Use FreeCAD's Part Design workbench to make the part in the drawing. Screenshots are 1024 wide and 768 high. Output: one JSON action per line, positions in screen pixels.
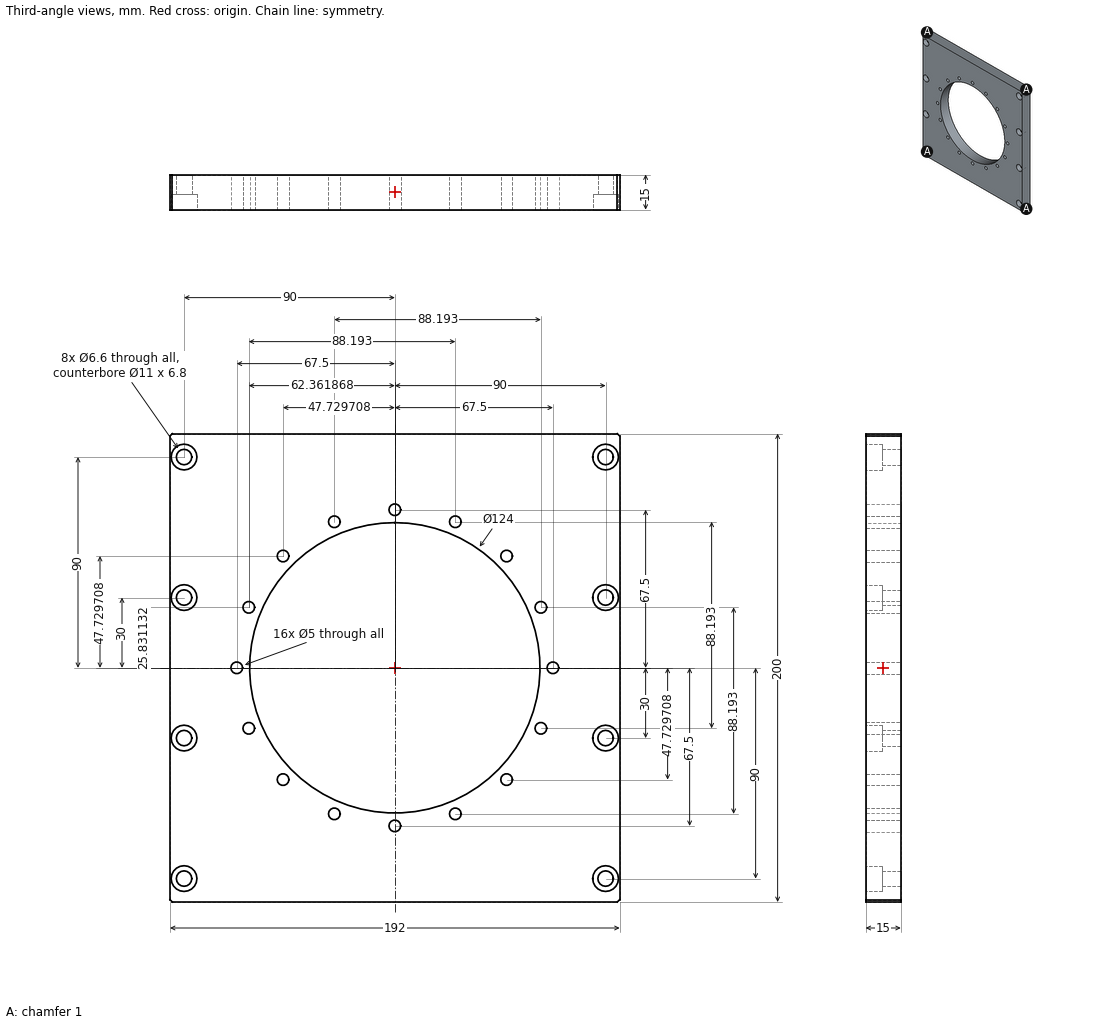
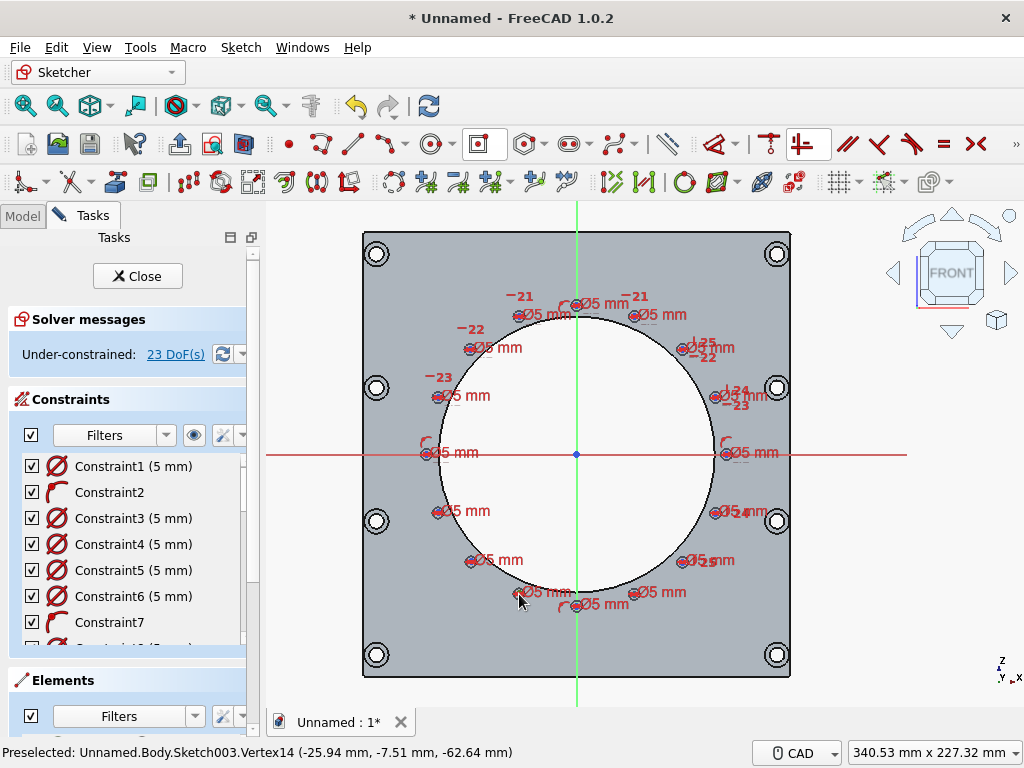
{"action": "key", "text": "h"}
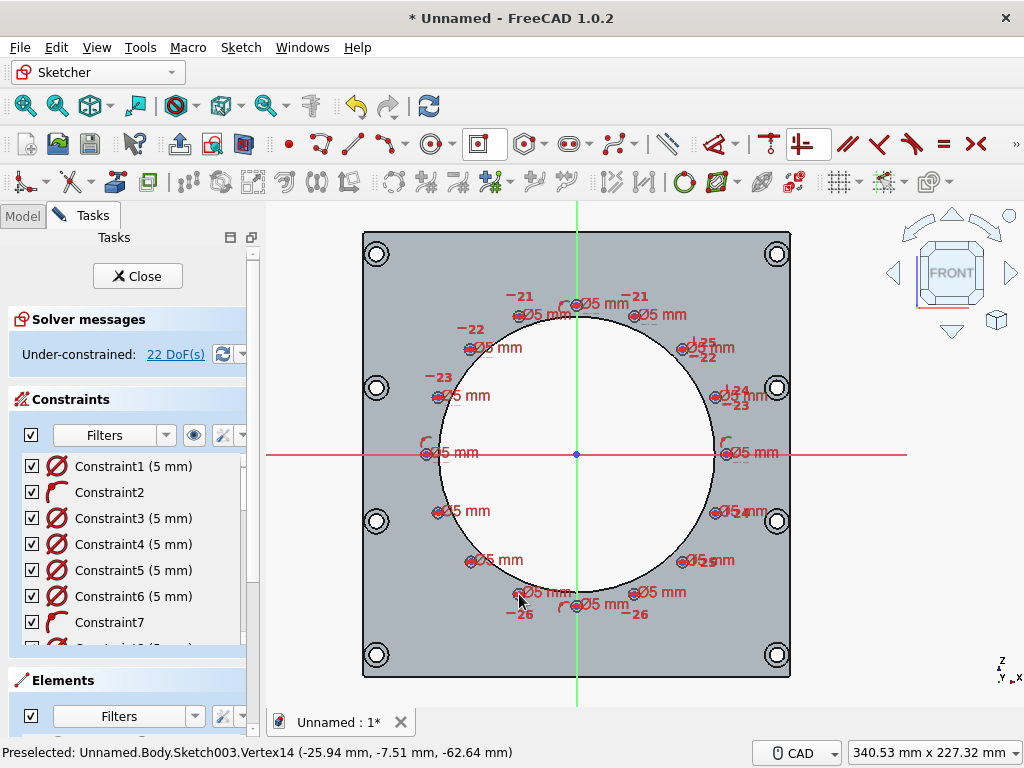
{"action": "left_click", "coordinate": [470, 350]}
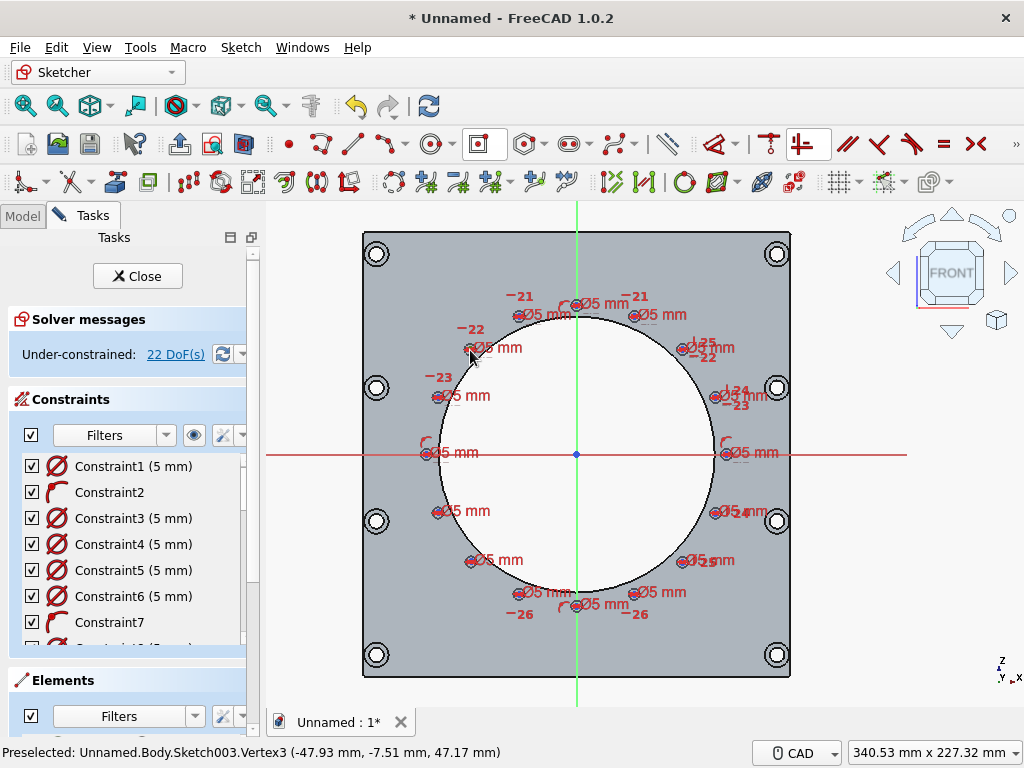
{"action": "left_click", "coordinate": [471, 562]}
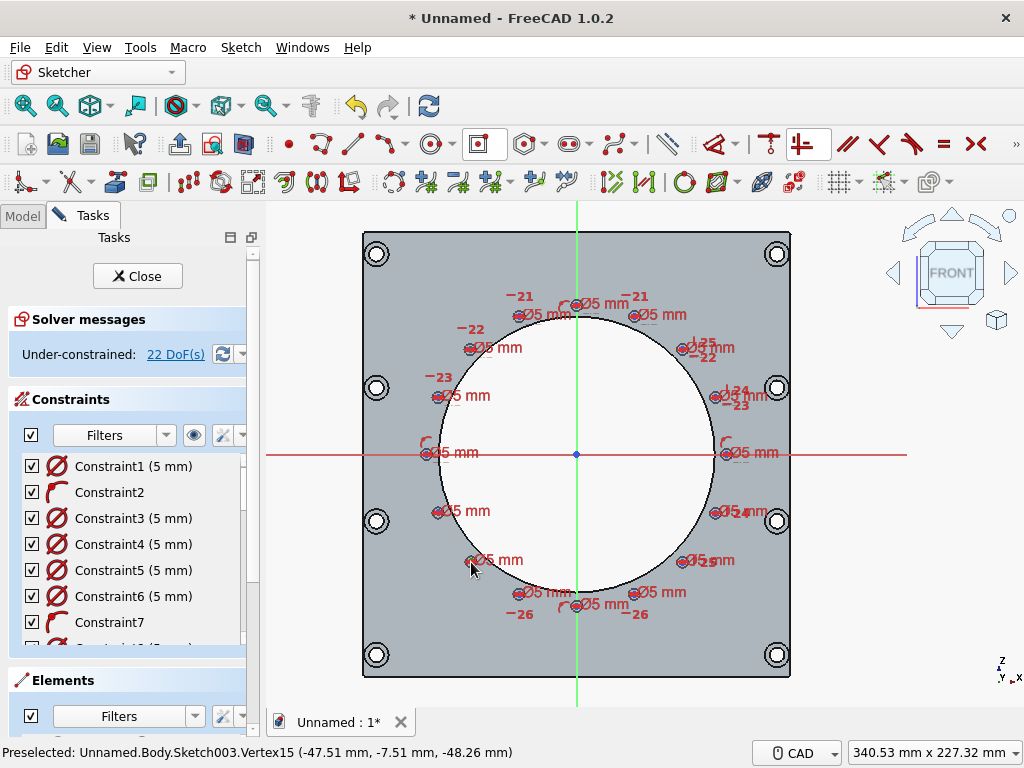
{"action": "left_click", "coordinate": [826, 144]}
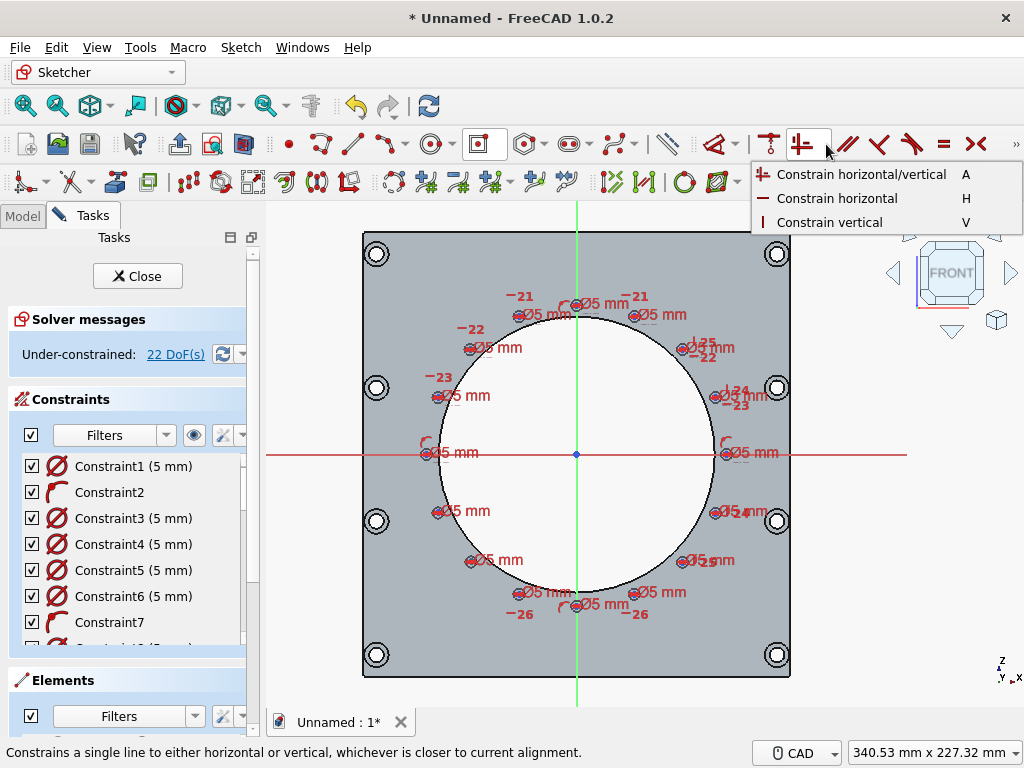
{"action": "left_click", "coordinate": [887, 222]}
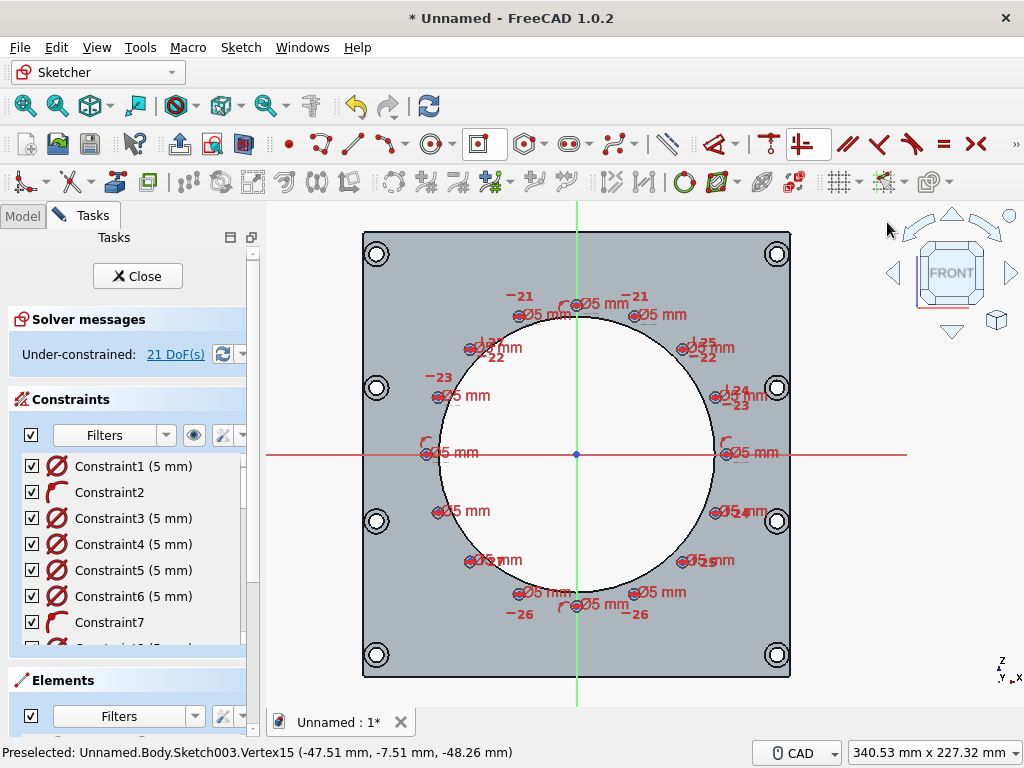
{"action": "left_click", "coordinate": [438, 398]}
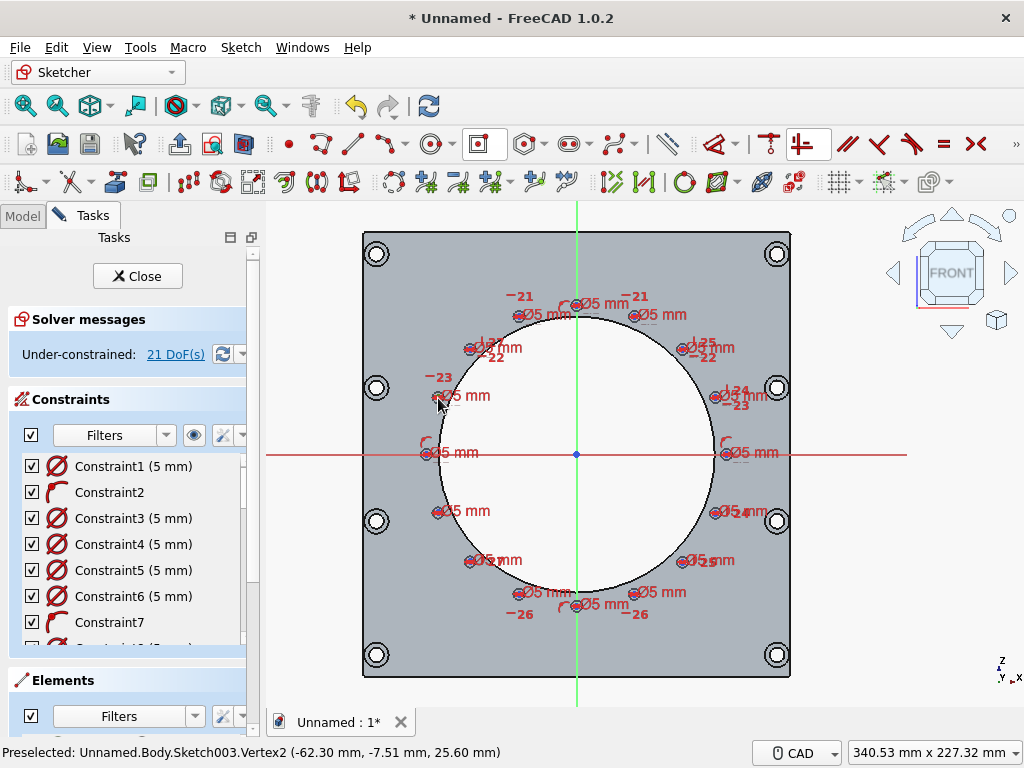
{"action": "left_click", "coordinate": [438, 513]}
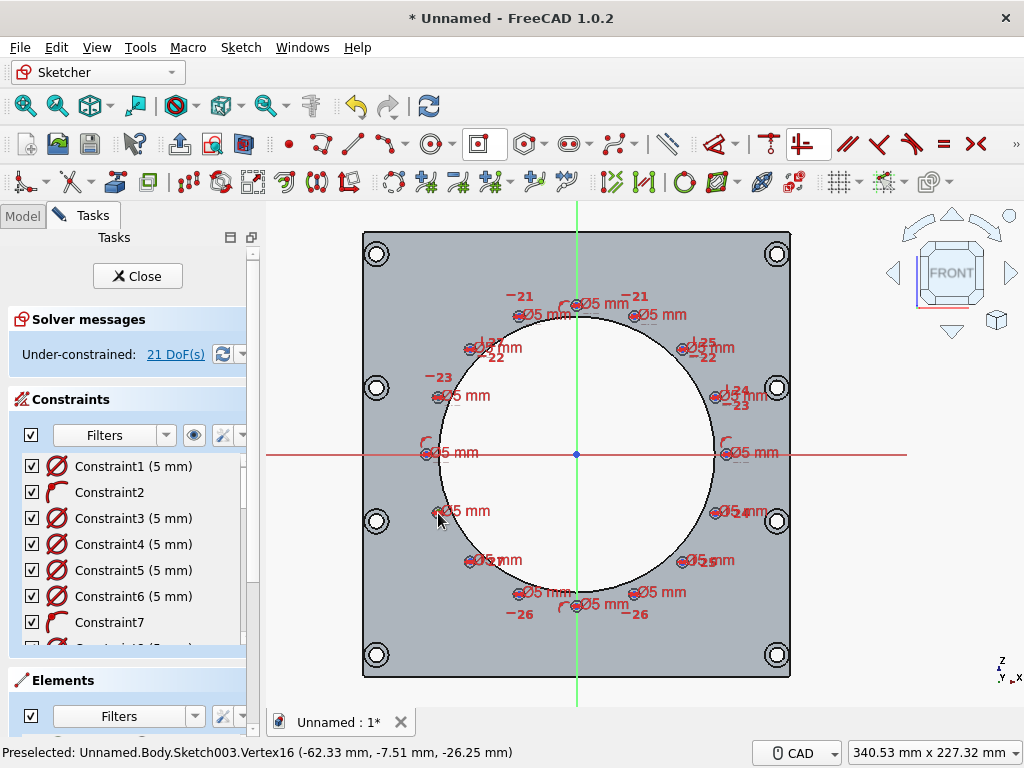
{"action": "left_click", "coordinate": [826, 144]}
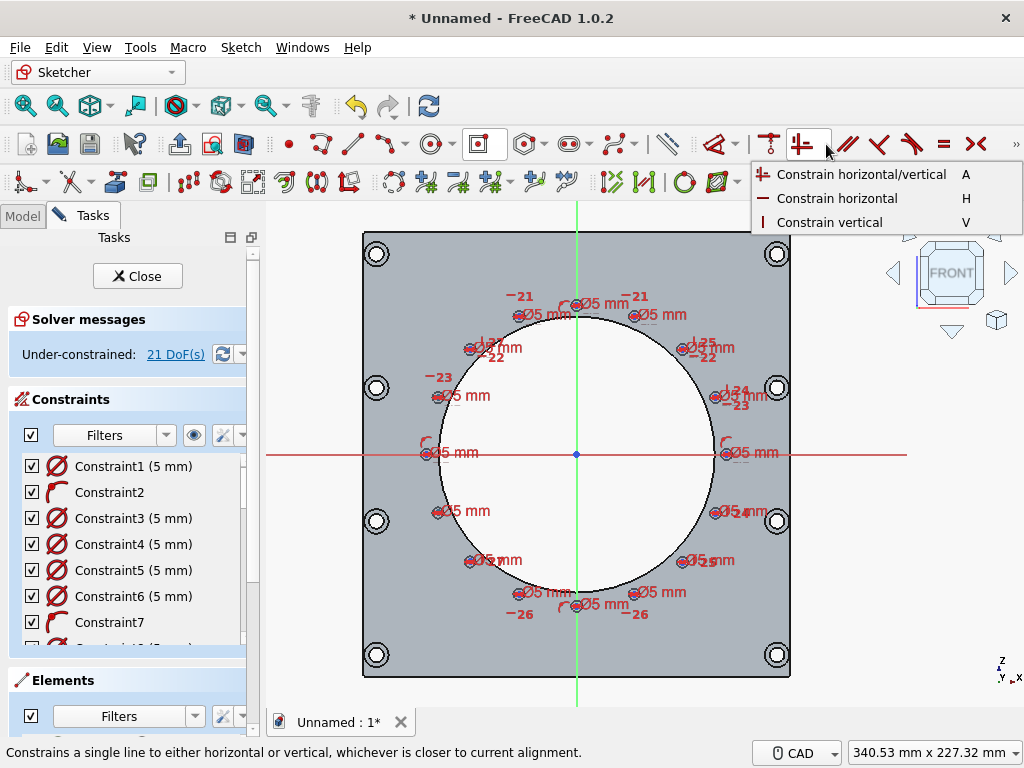
{"action": "left_click", "coordinate": [887, 222]}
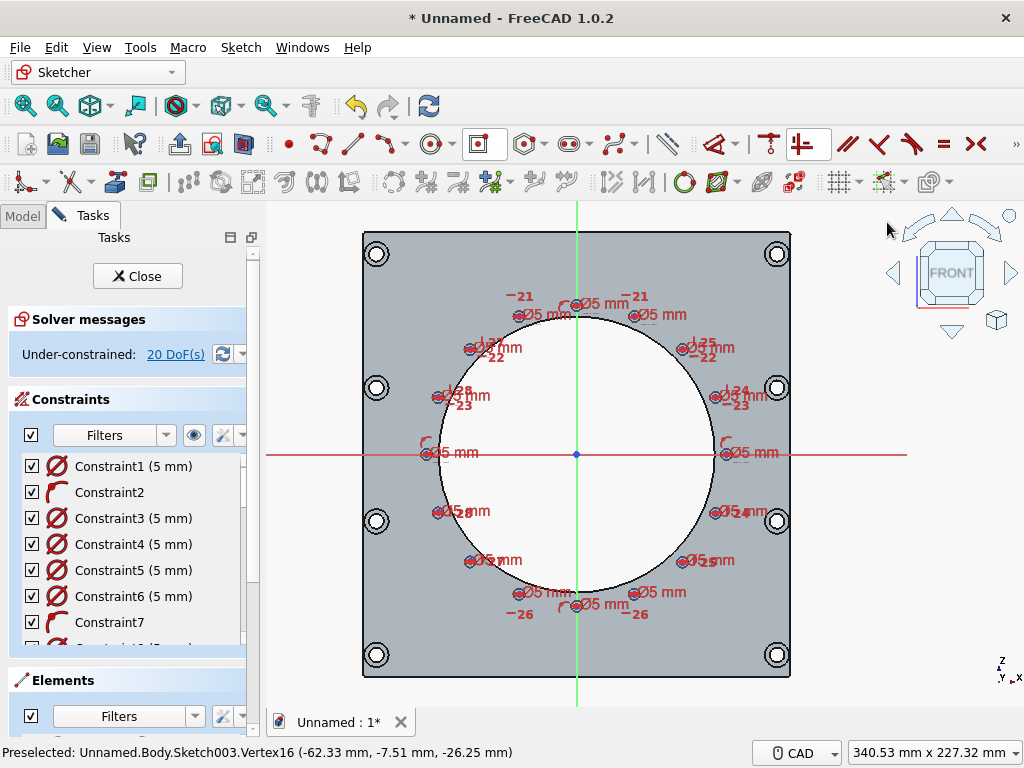
{"action": "left_click", "coordinate": [635, 317]}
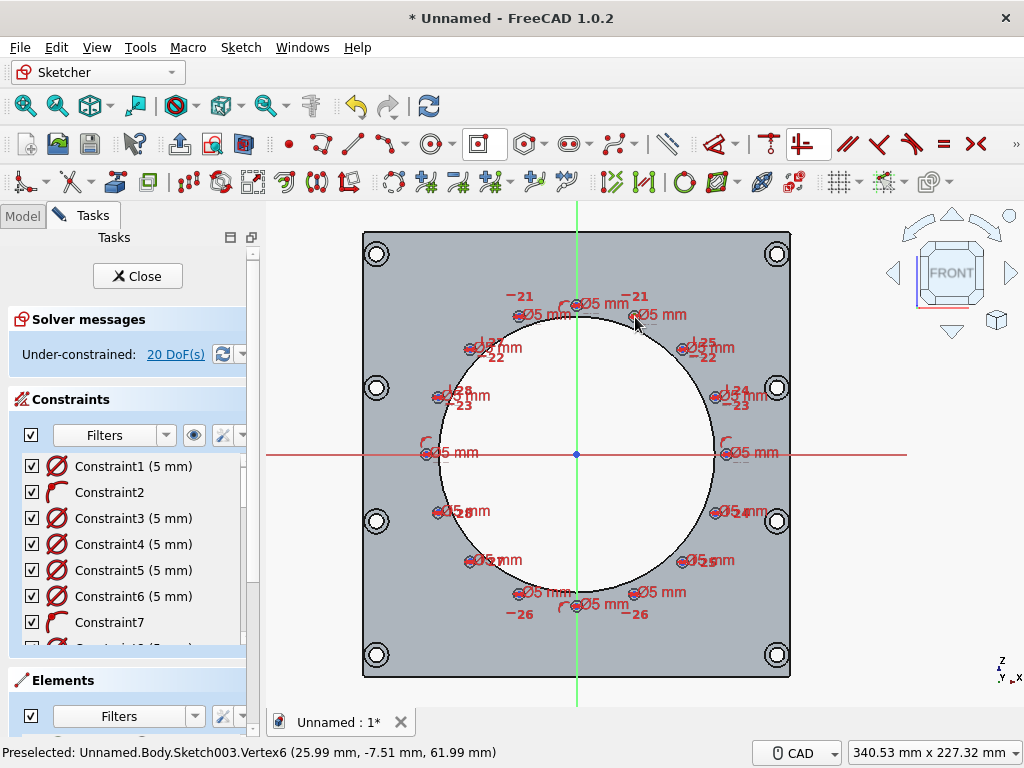
{"action": "left_click", "coordinate": [634, 594]}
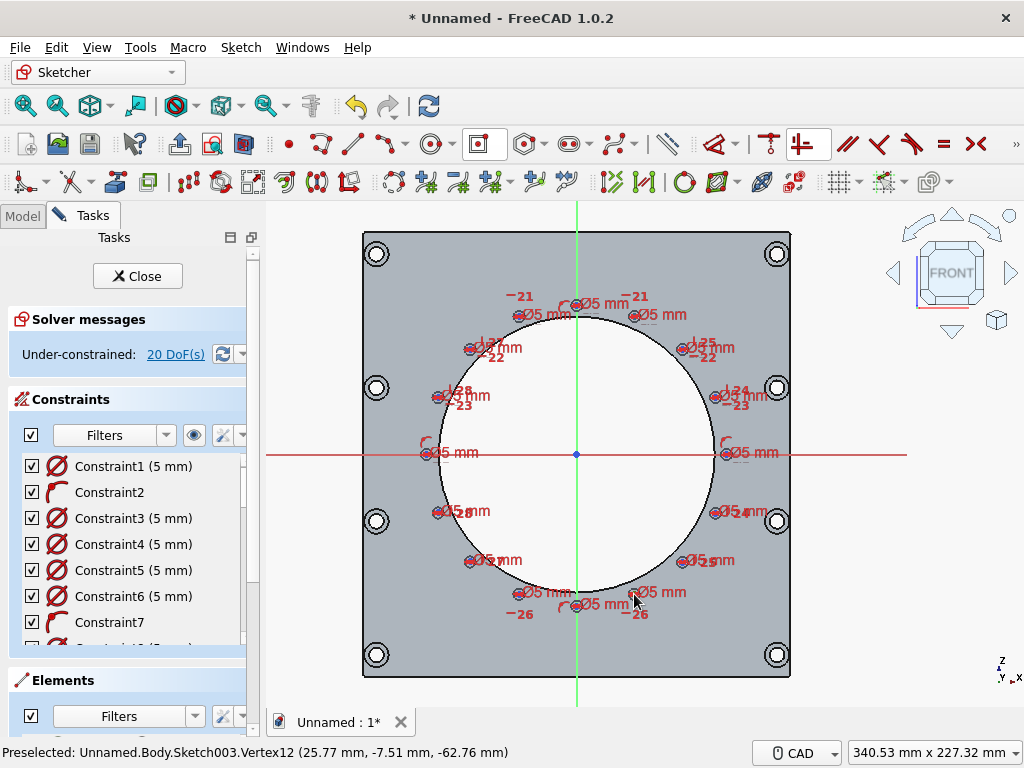
{"action": "left_click", "coordinate": [334, 455]}